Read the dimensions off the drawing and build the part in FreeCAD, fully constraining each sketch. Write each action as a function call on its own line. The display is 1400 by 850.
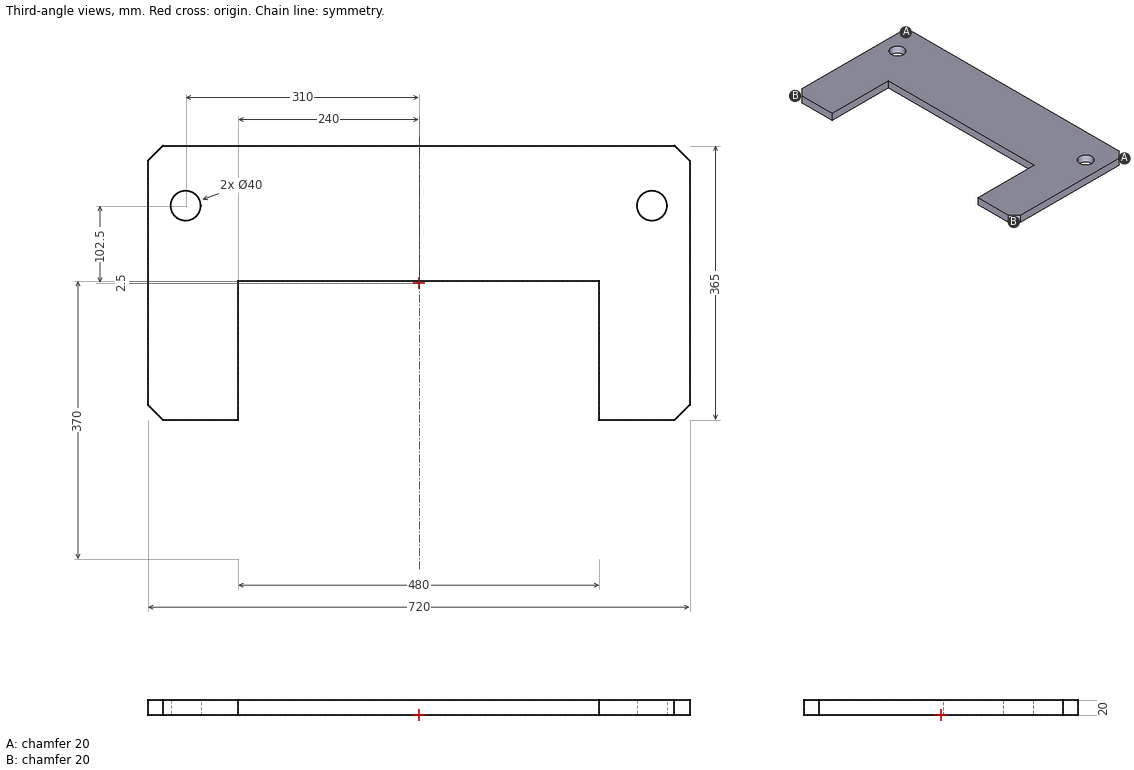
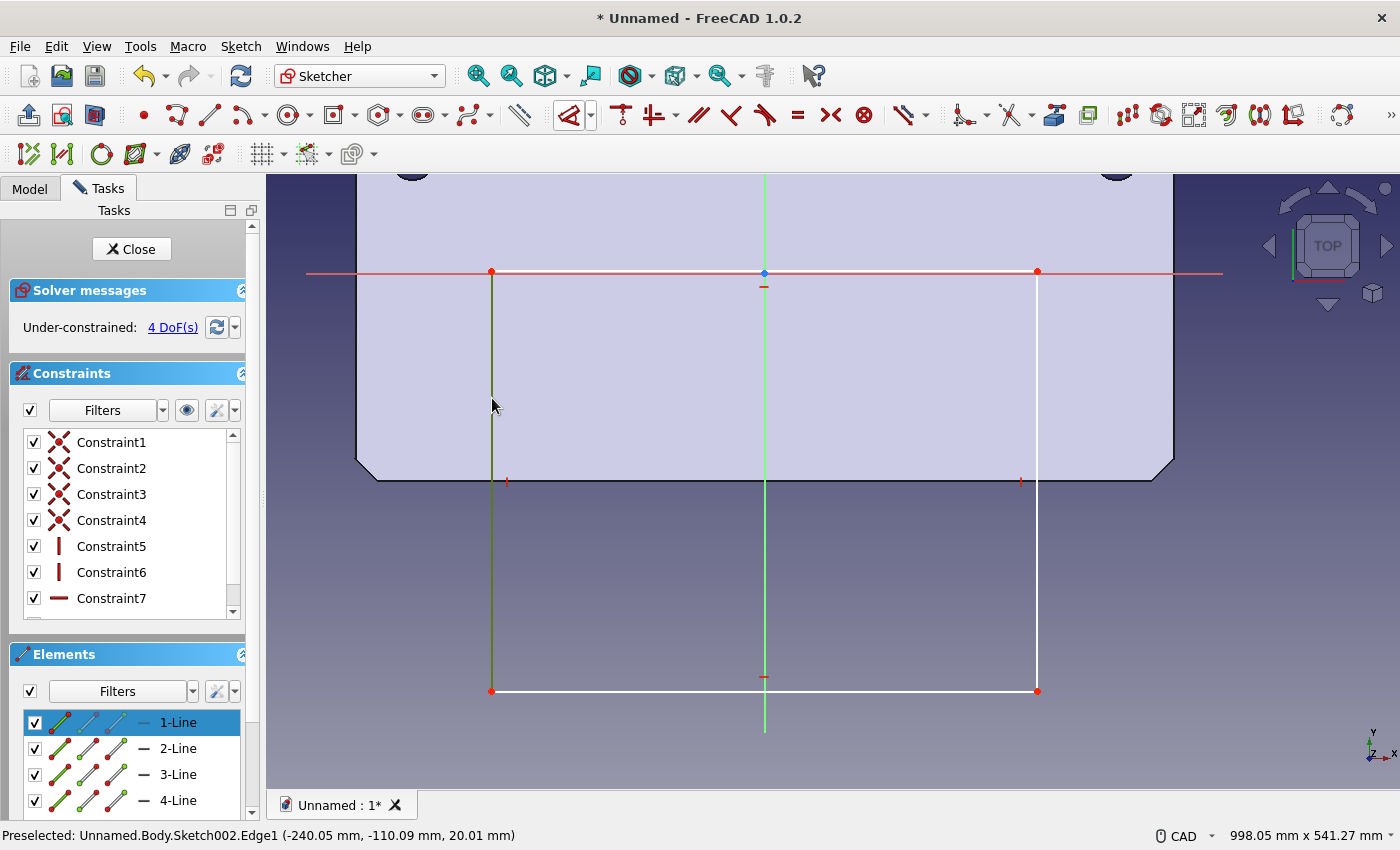
click(590, 116)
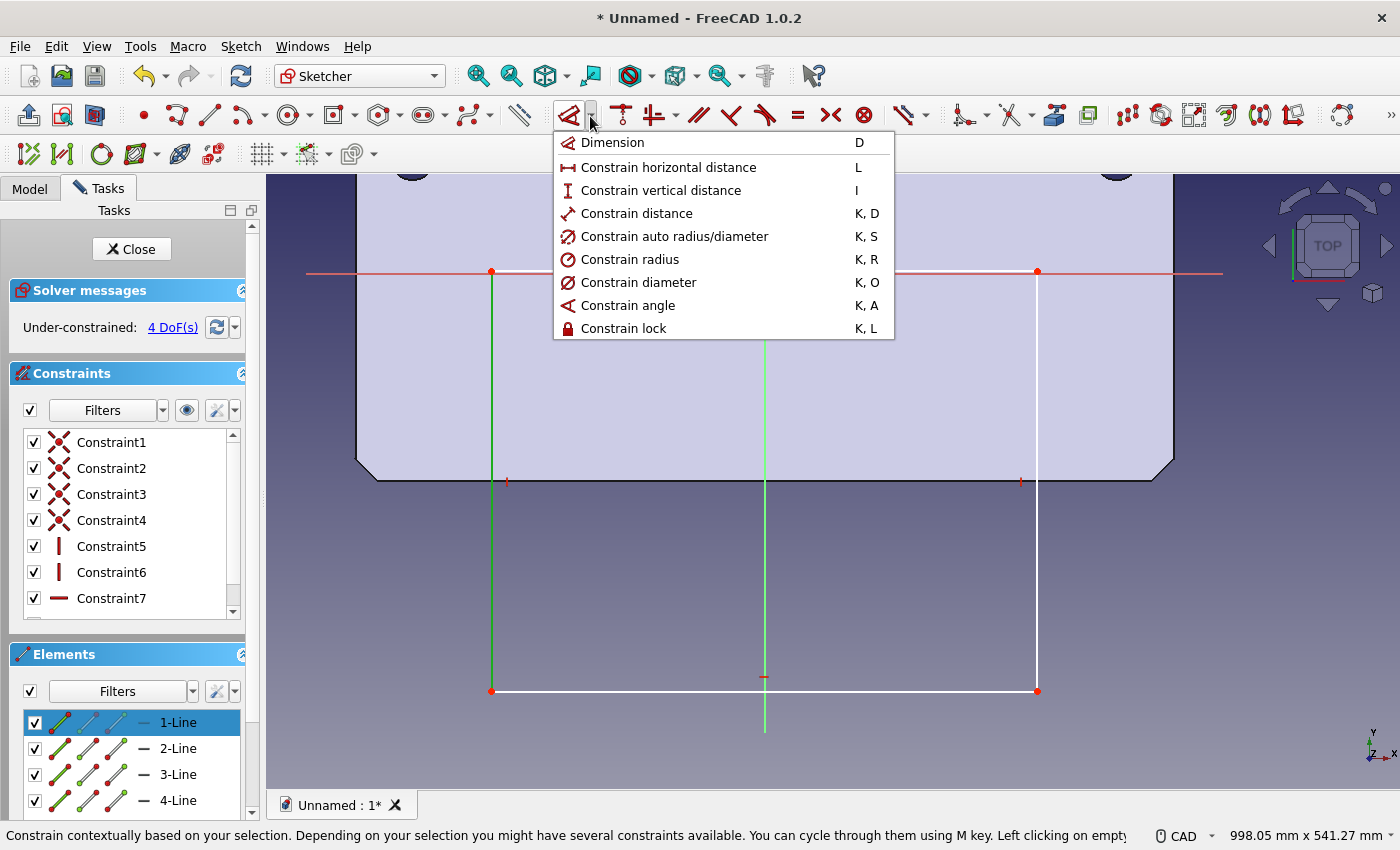
click(724, 190)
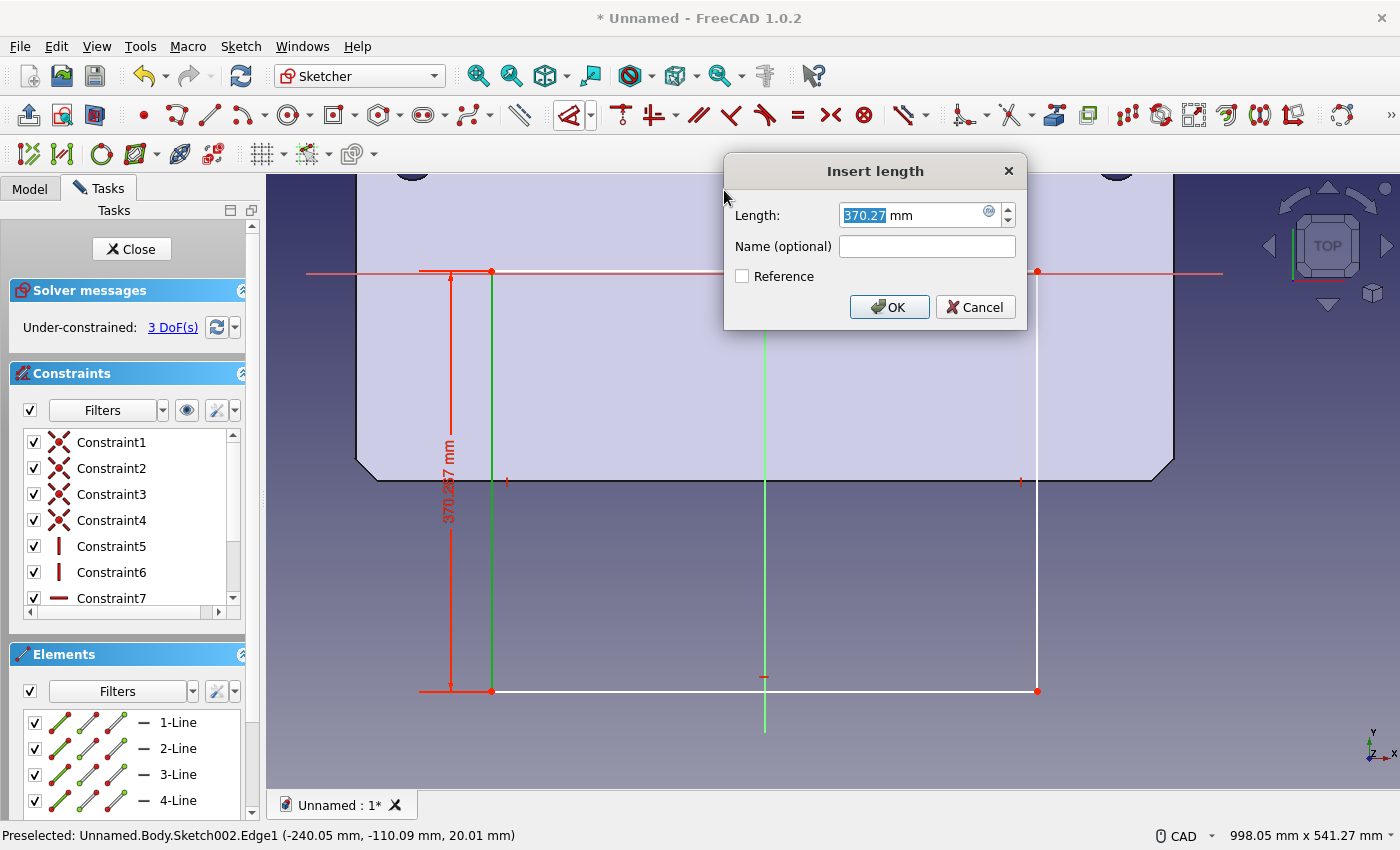
text(370)
key(Return)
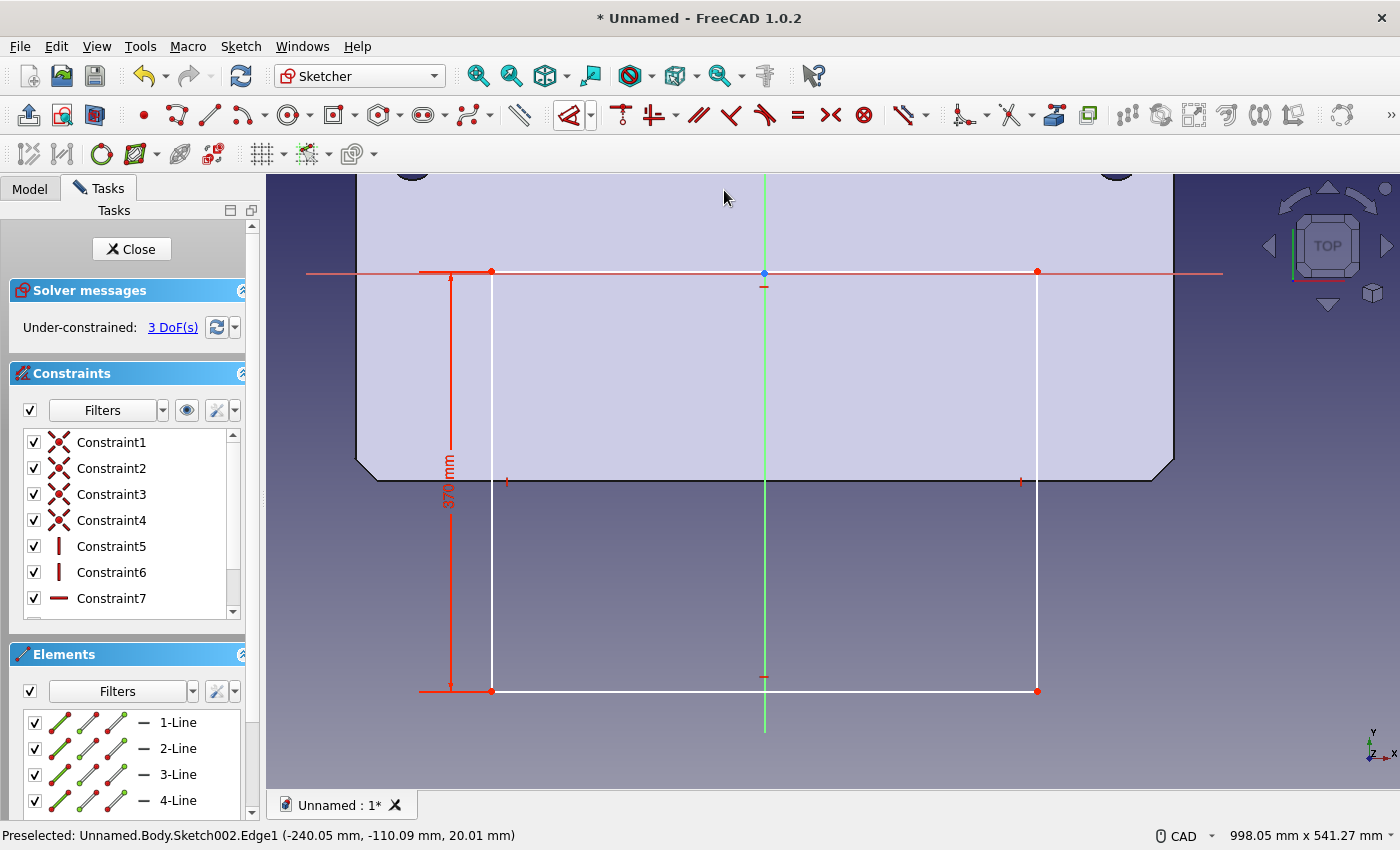
click(655, 692)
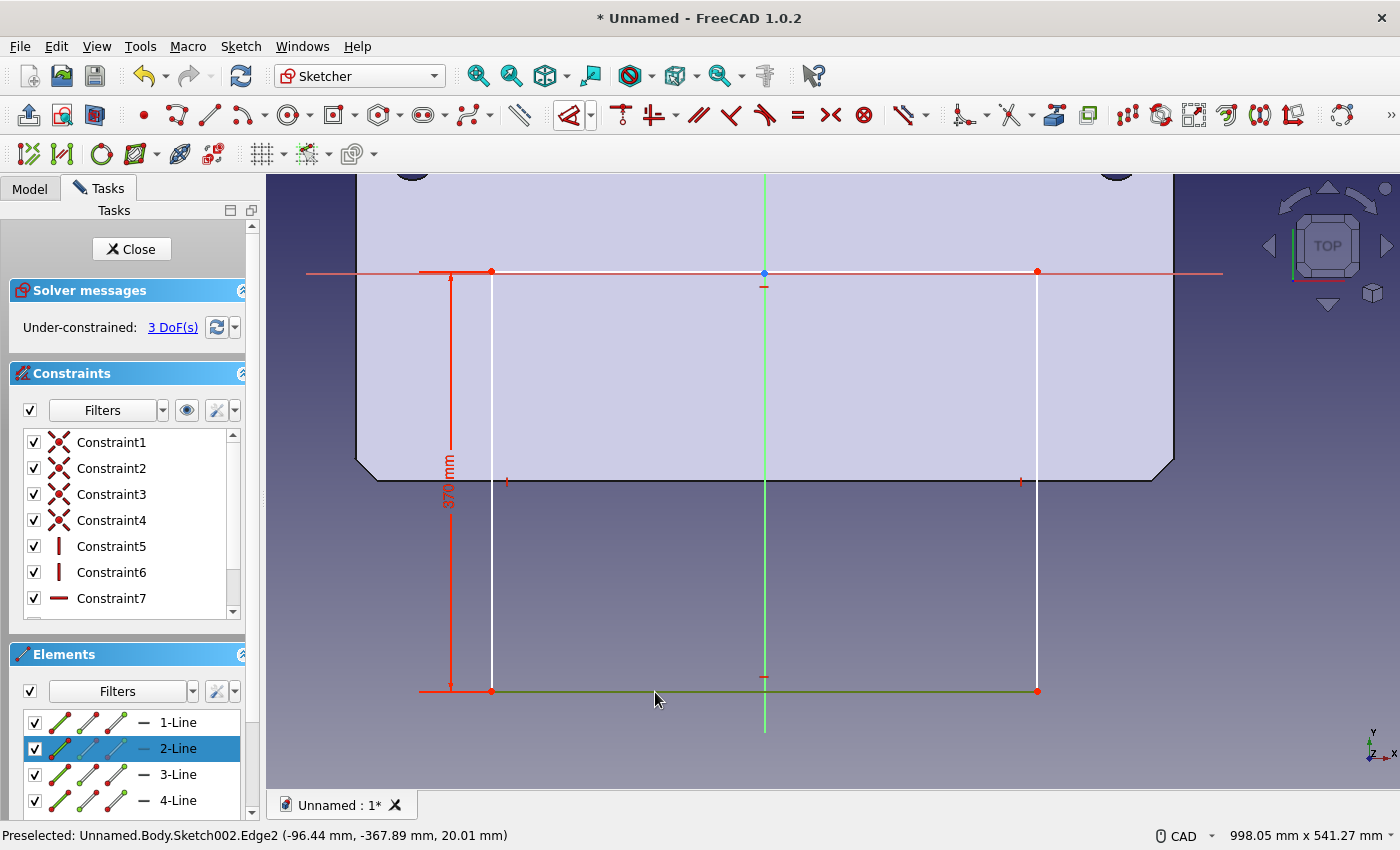
key(l)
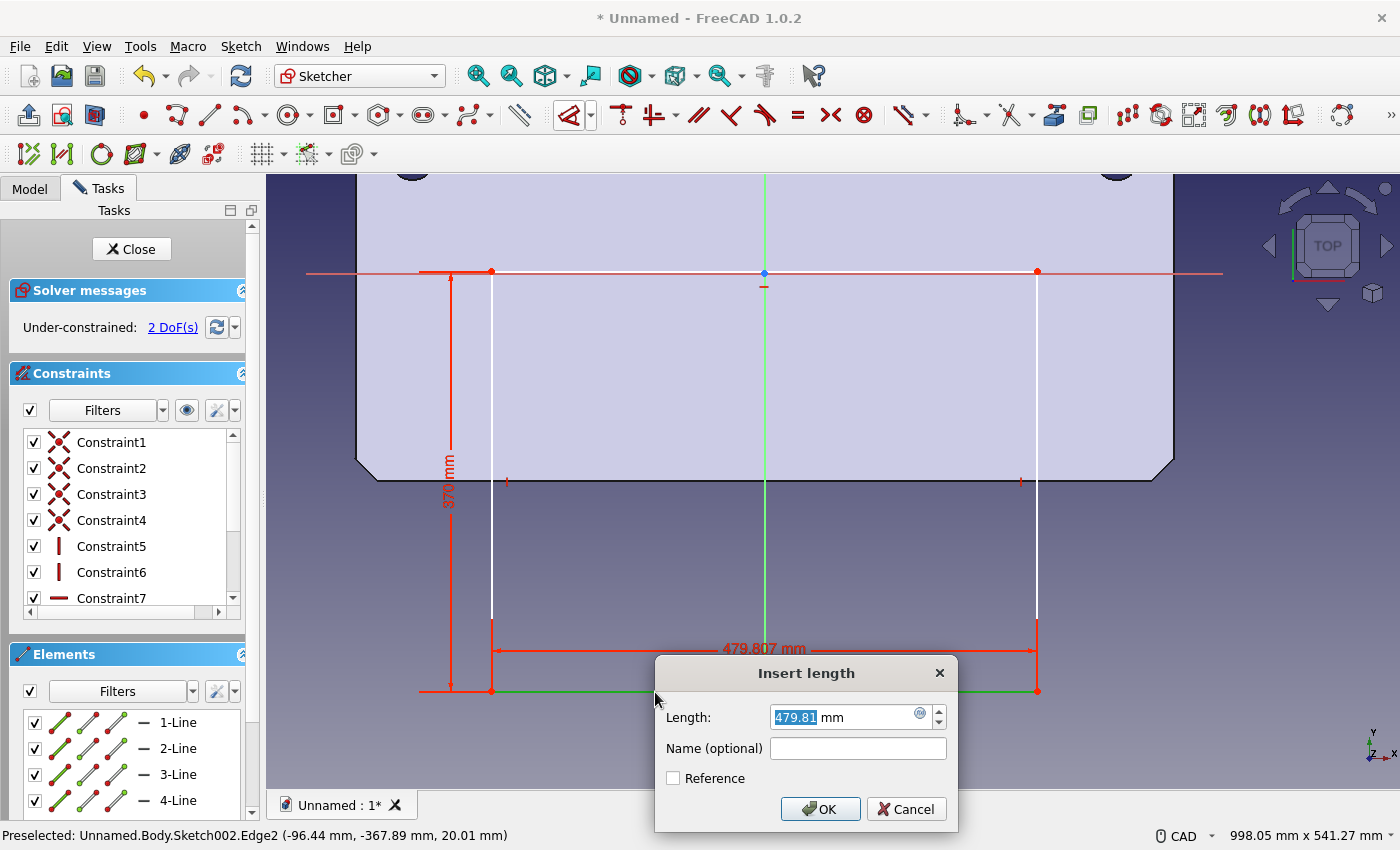
text(480)
key(Return)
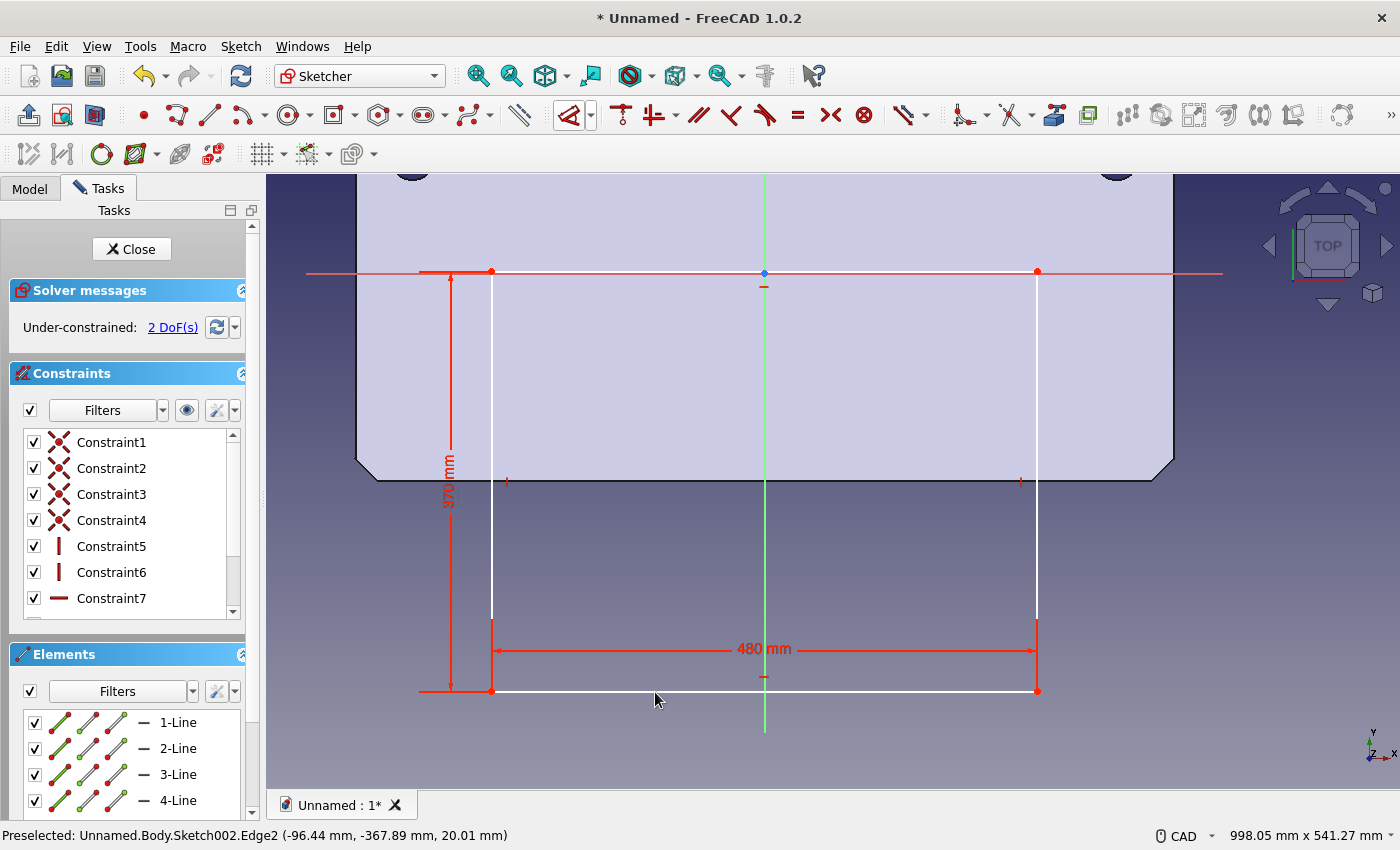
click(492, 272)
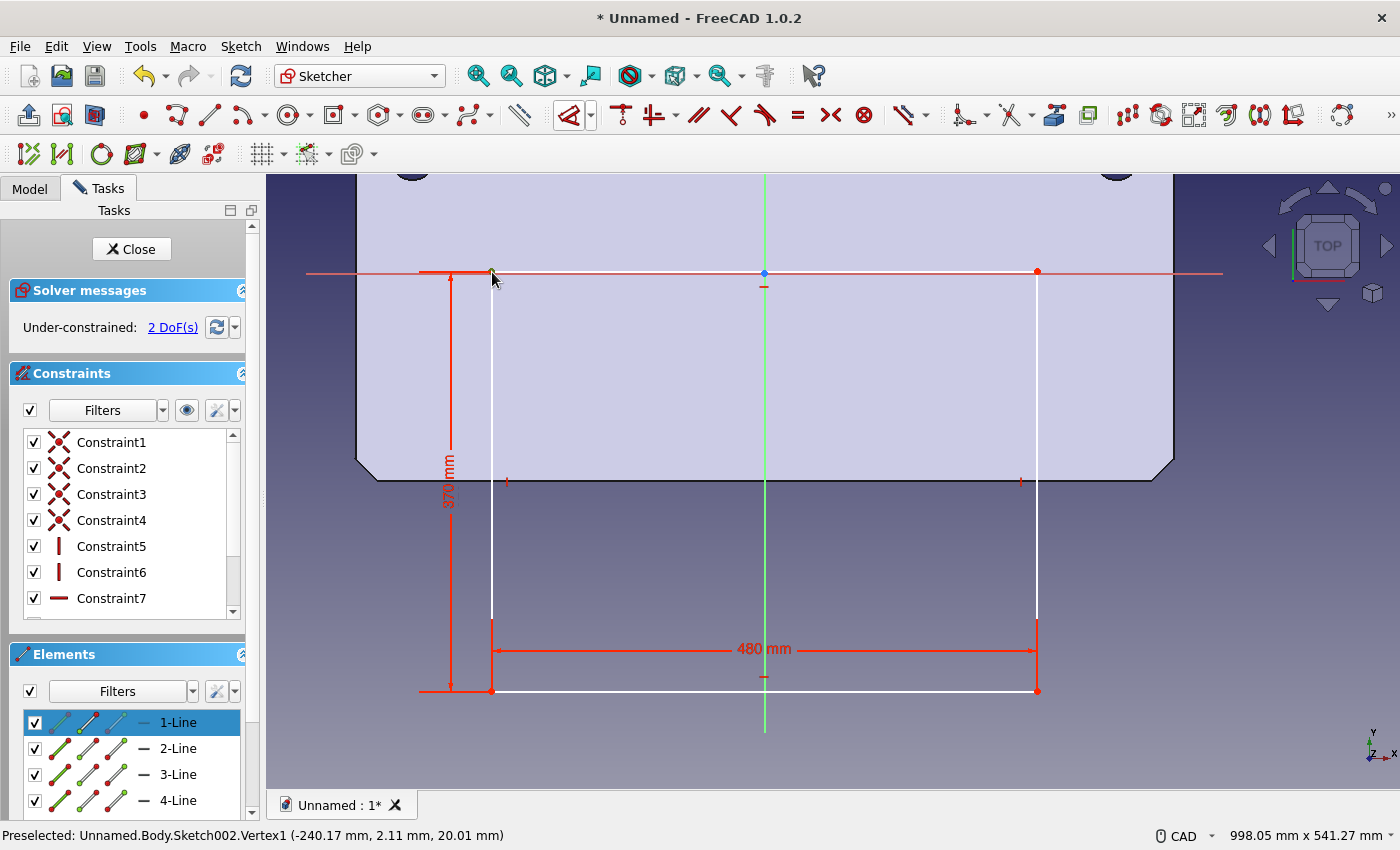
key(l)